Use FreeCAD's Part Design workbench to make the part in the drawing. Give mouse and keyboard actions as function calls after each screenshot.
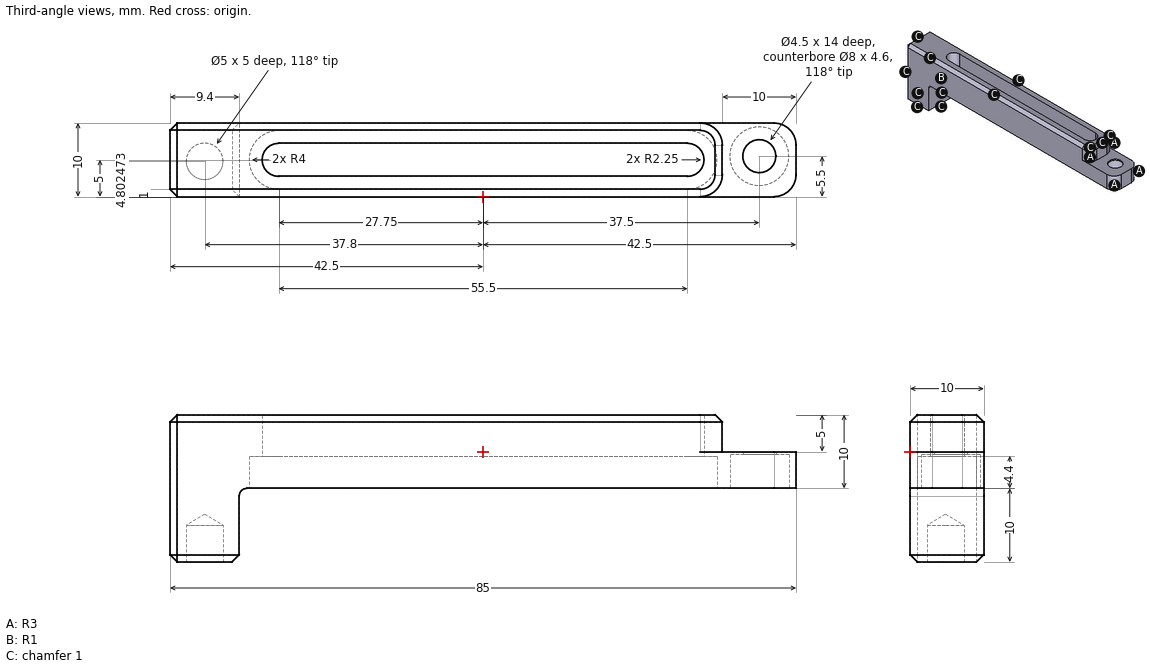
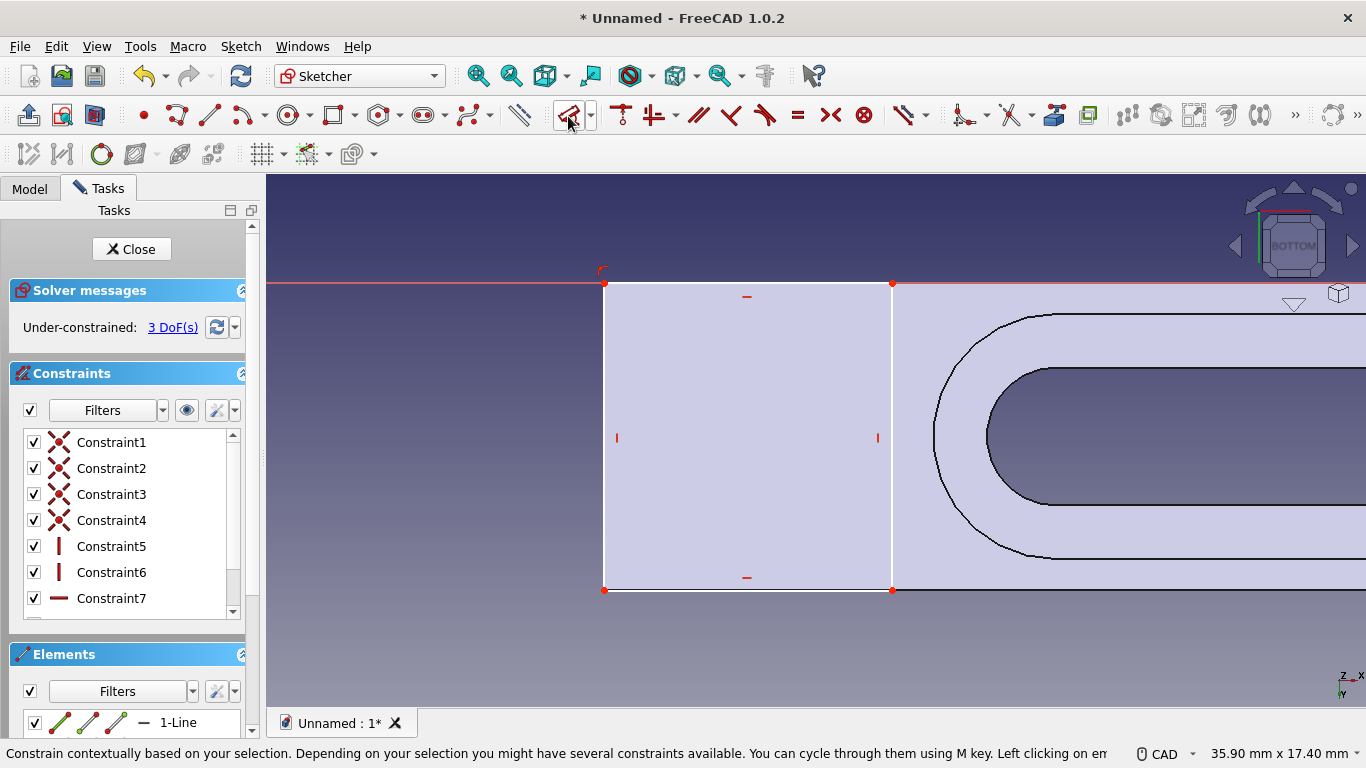
click(604, 376)
click(570, 437)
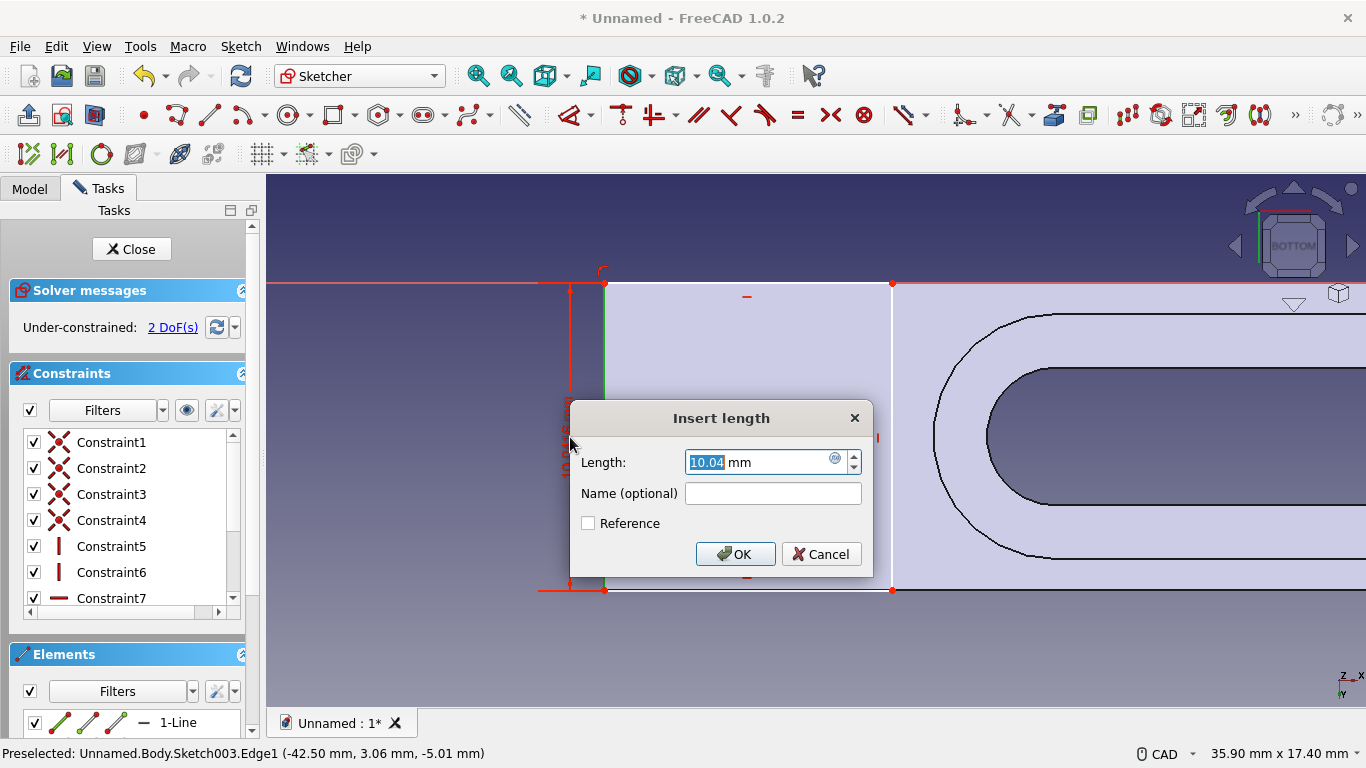
text(10)
key(Return)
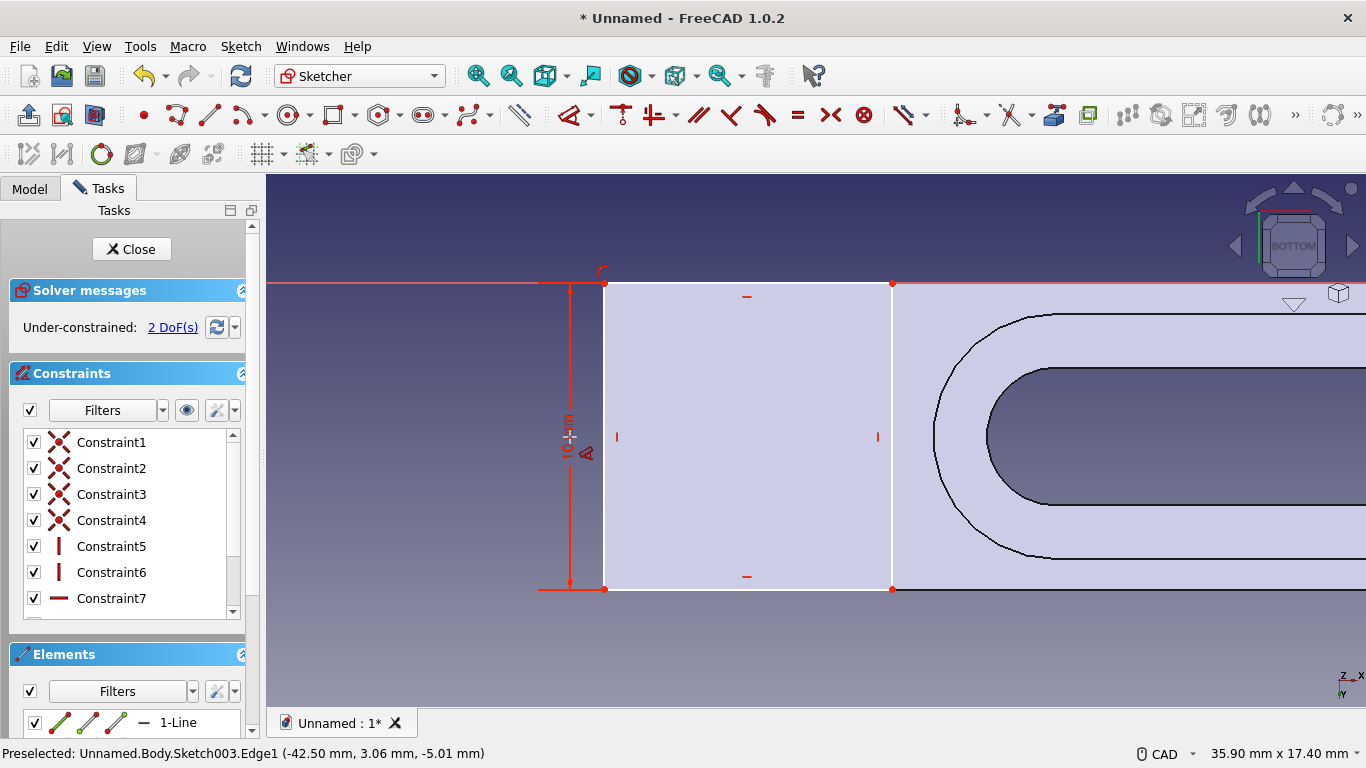
click(690, 590)
click(748, 624)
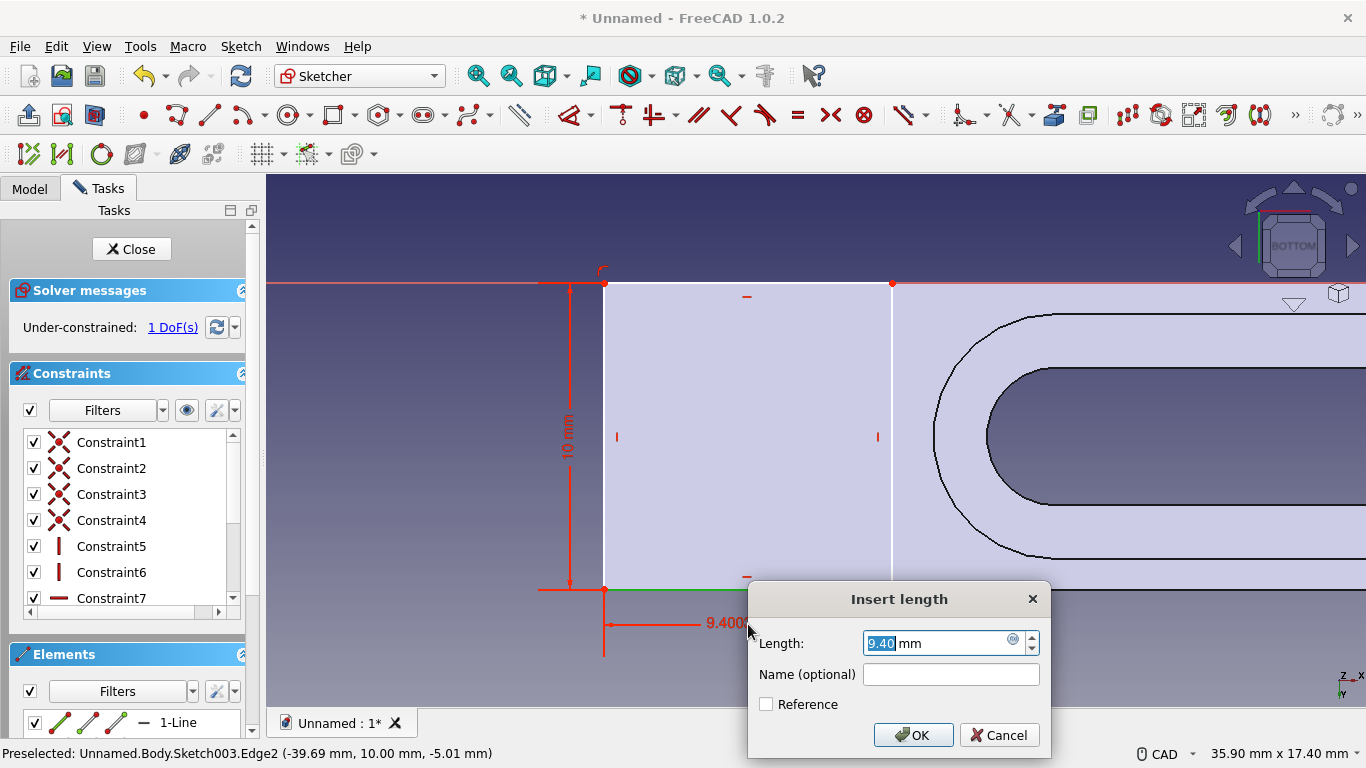
text(9.4)
key(Return)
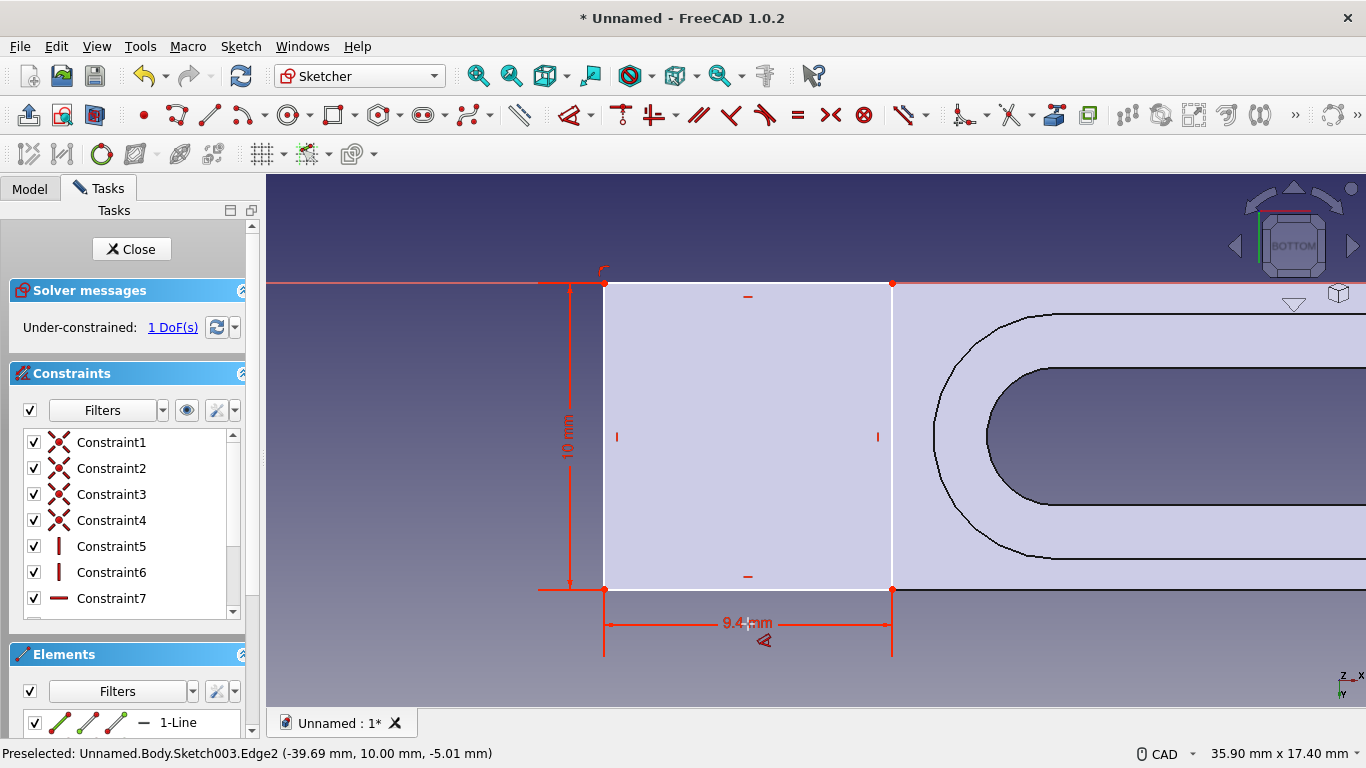
click(604, 283)
click(903, 249)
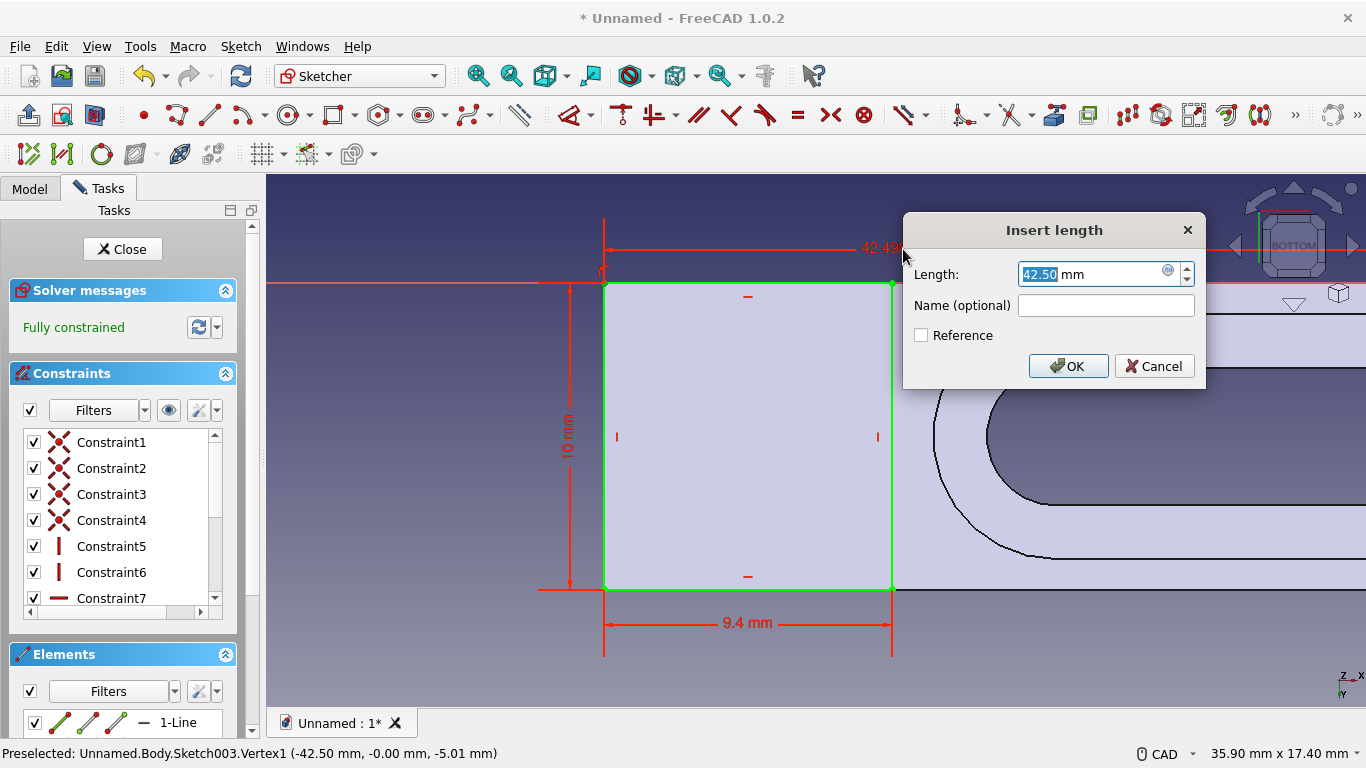
text(42.5)
key(Return)
key(Escape)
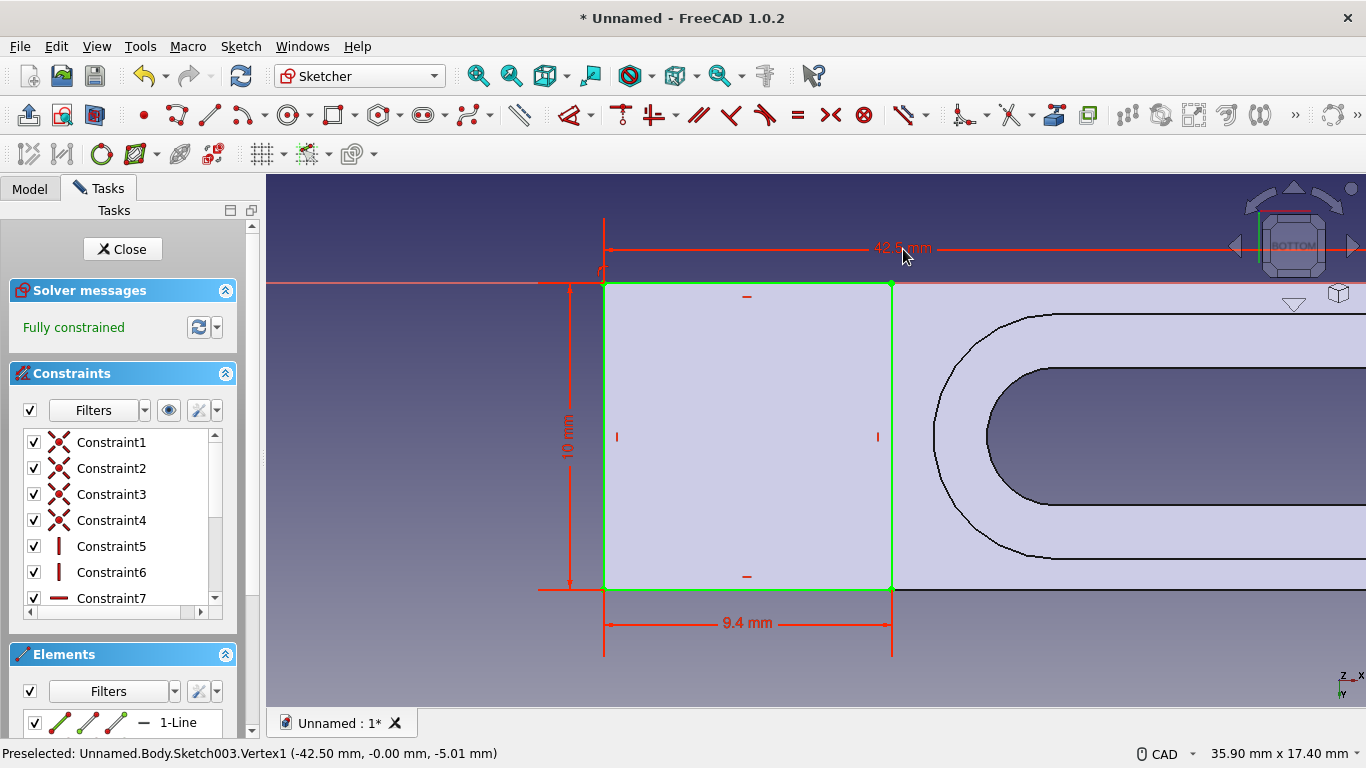
click(123, 249)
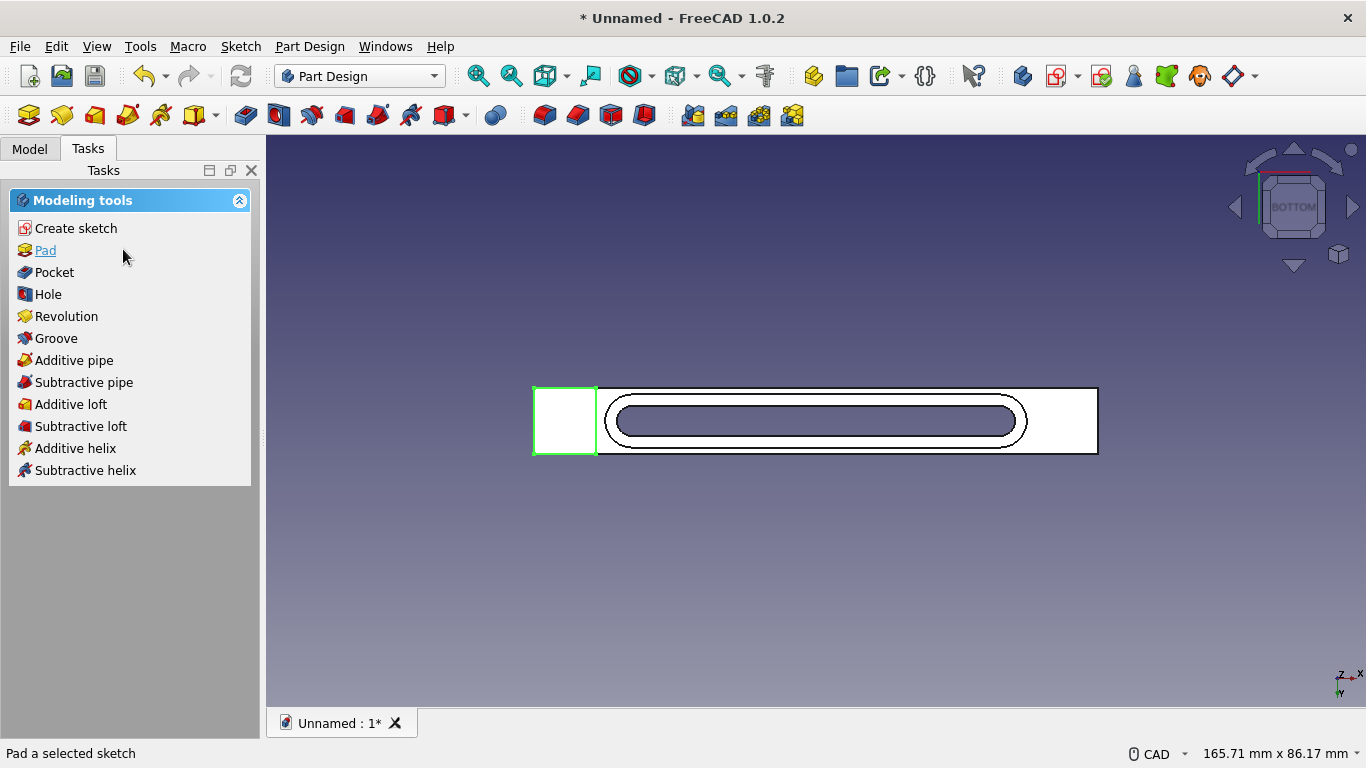
click(29, 116)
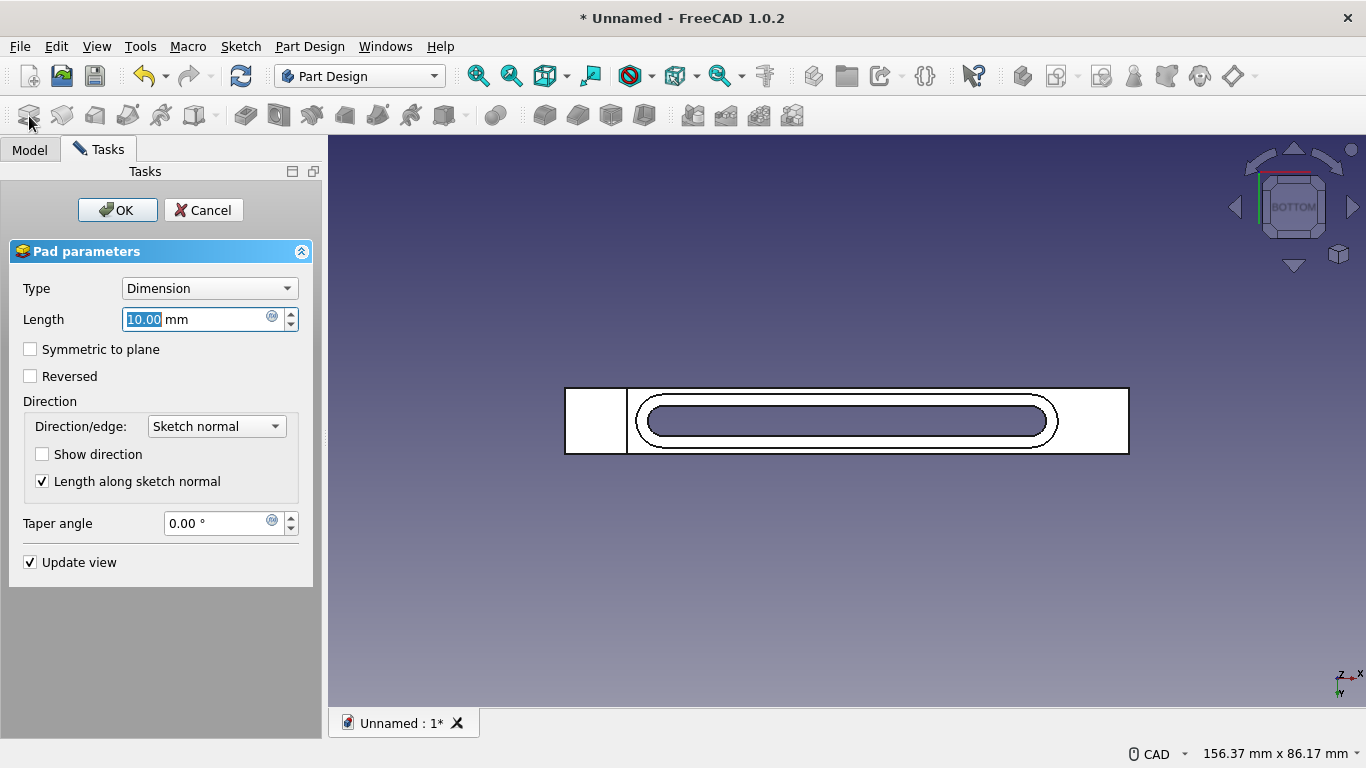
text(10)
key(Tab)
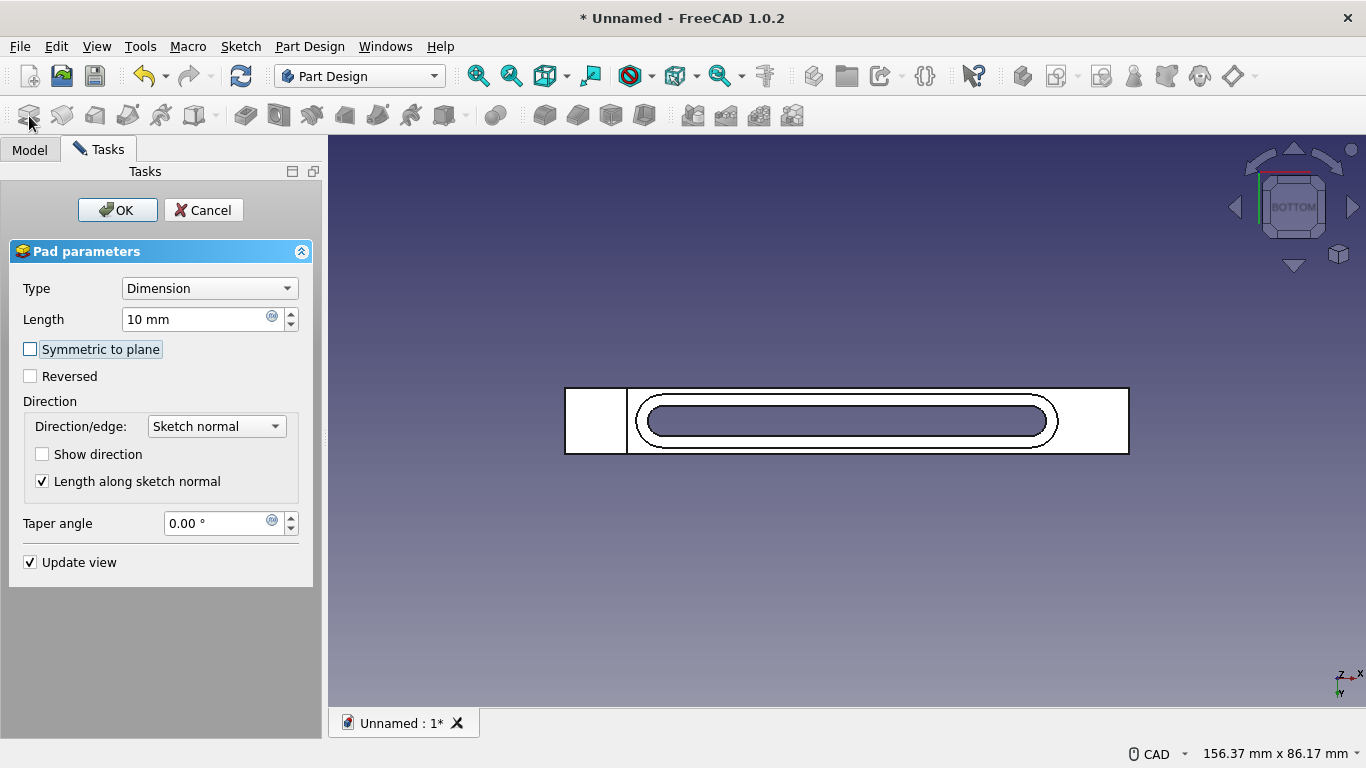
click(118, 210)